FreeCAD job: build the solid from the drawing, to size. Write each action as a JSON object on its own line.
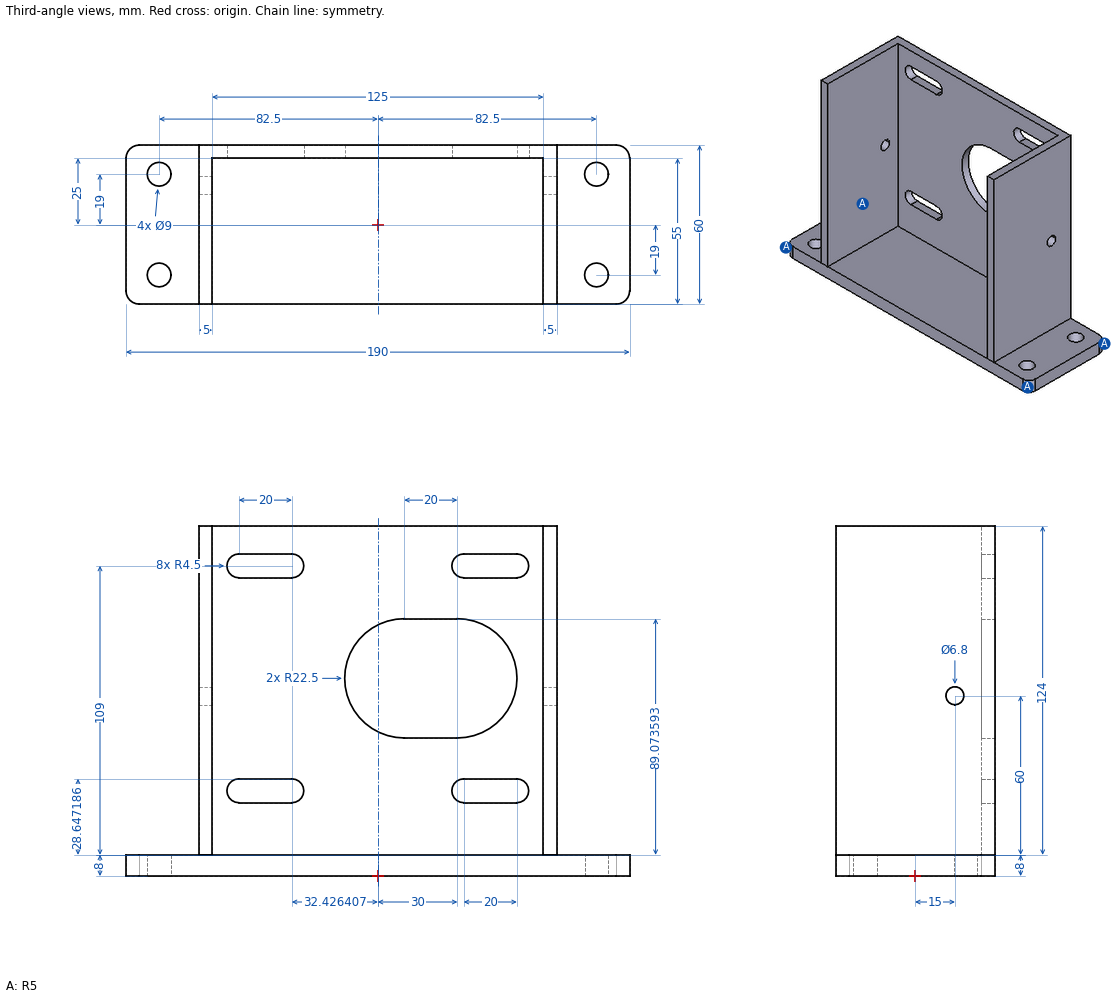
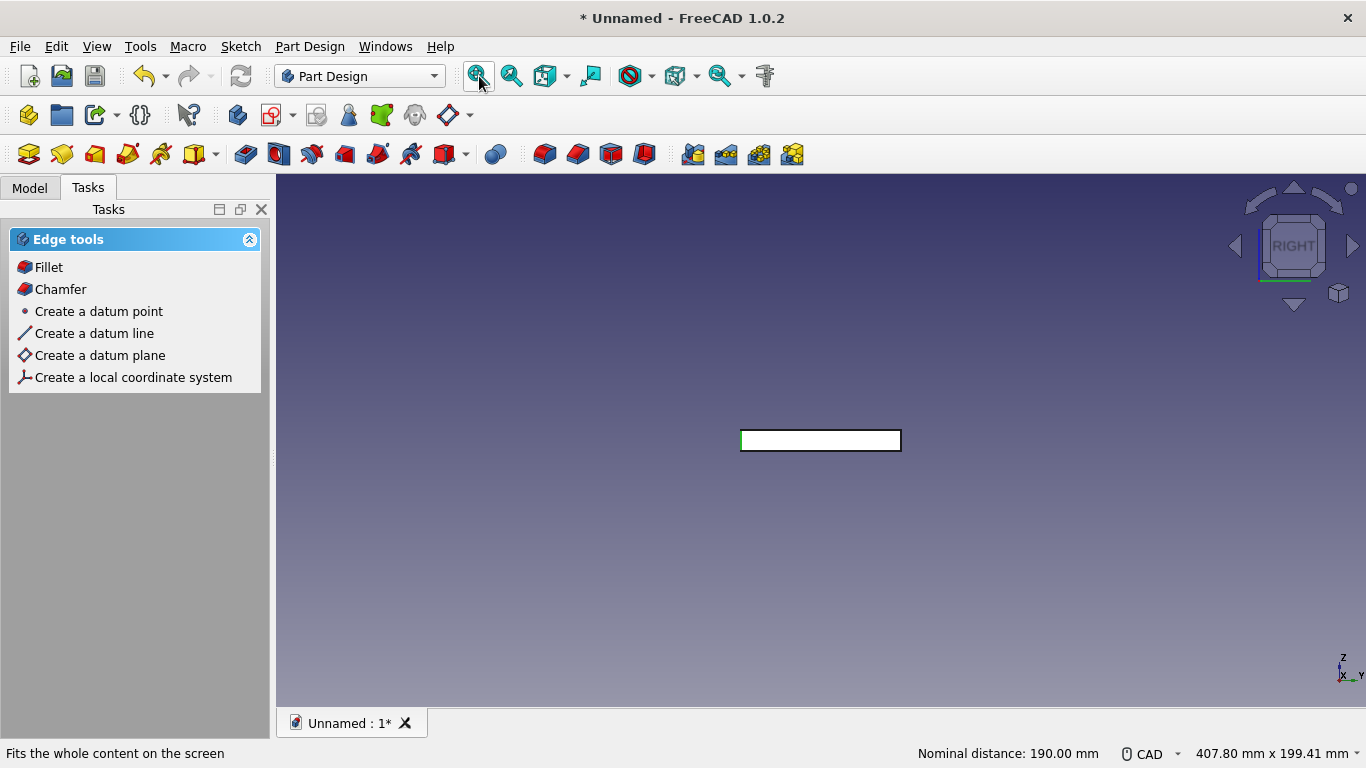
{"action": "left_click", "coordinate": [901, 439], "text": "ctrl"}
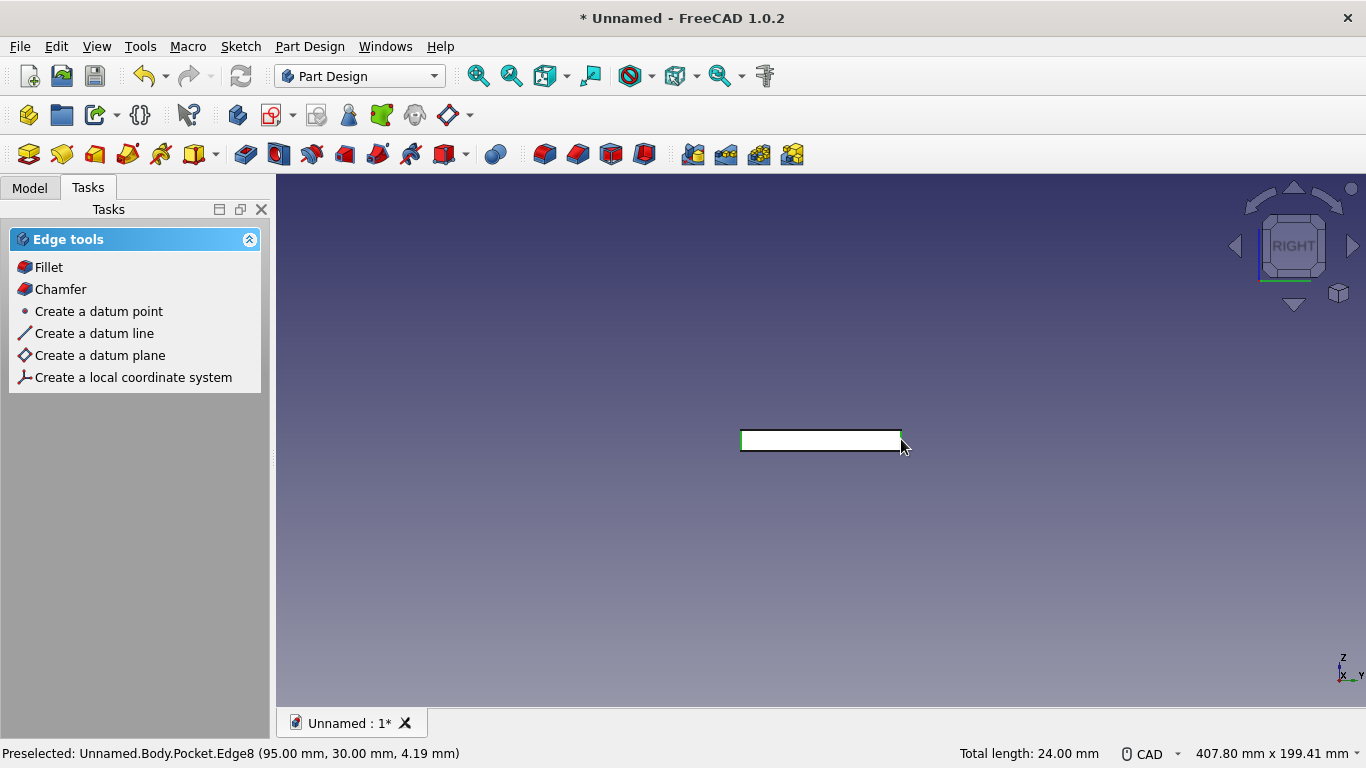
{"action": "scroll", "coordinate": [901, 439], "scroll_direction": "up", "scroll_amount": 4}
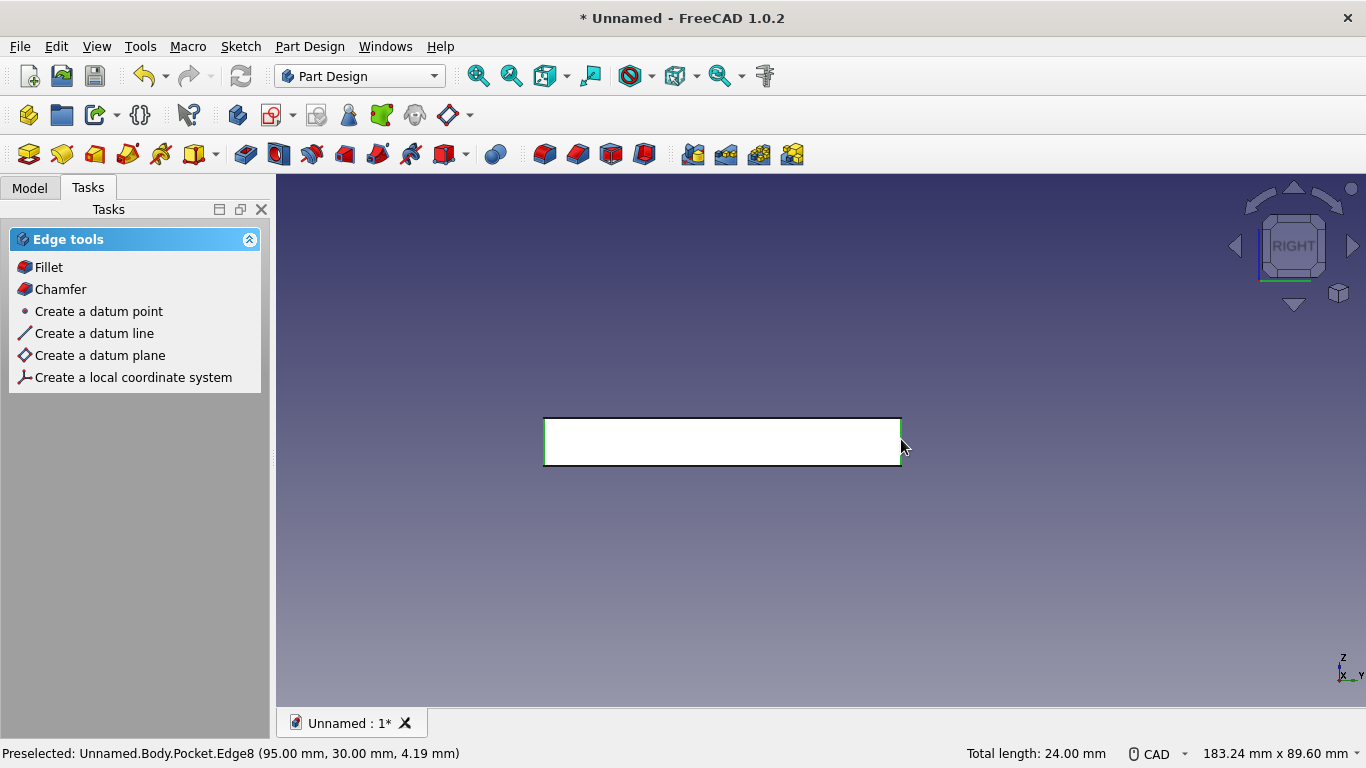
{"action": "left_click", "coordinate": [479, 76]}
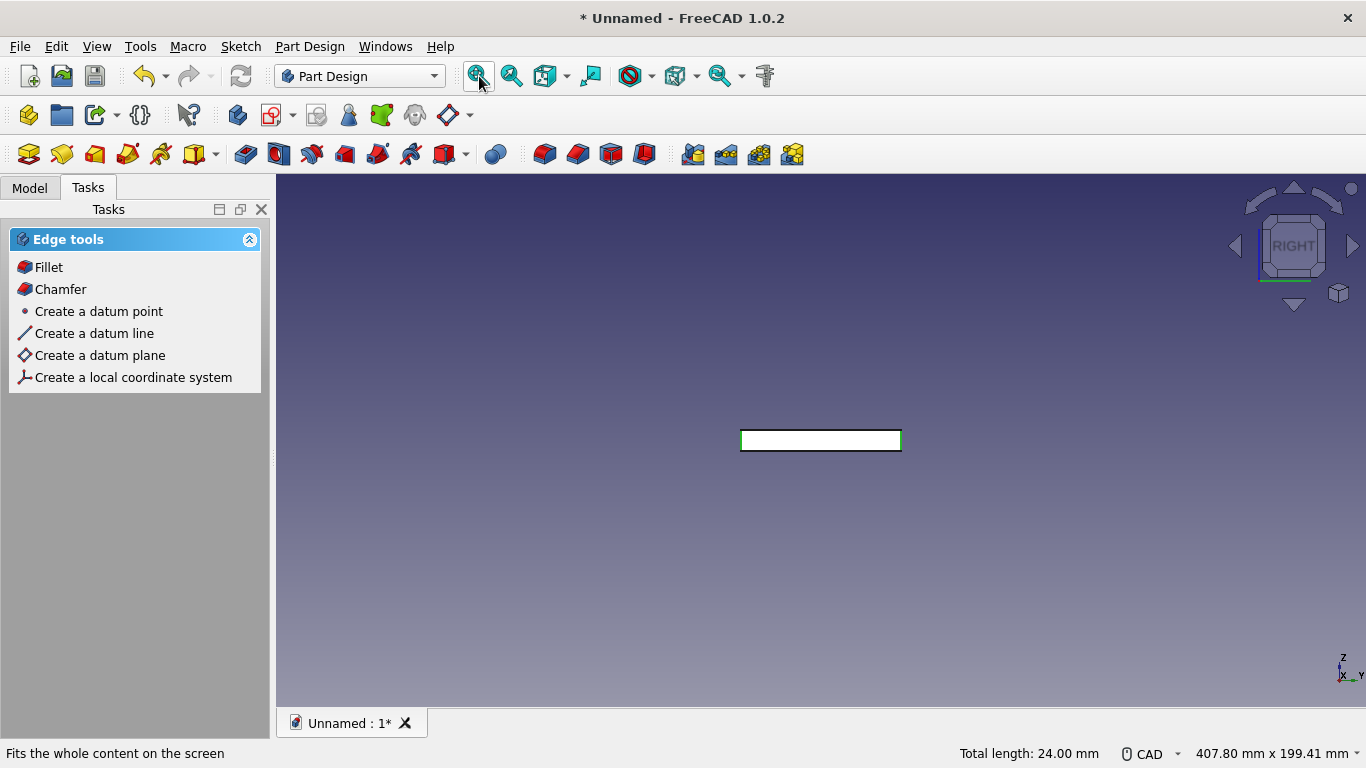
{"action": "key", "text": "5"}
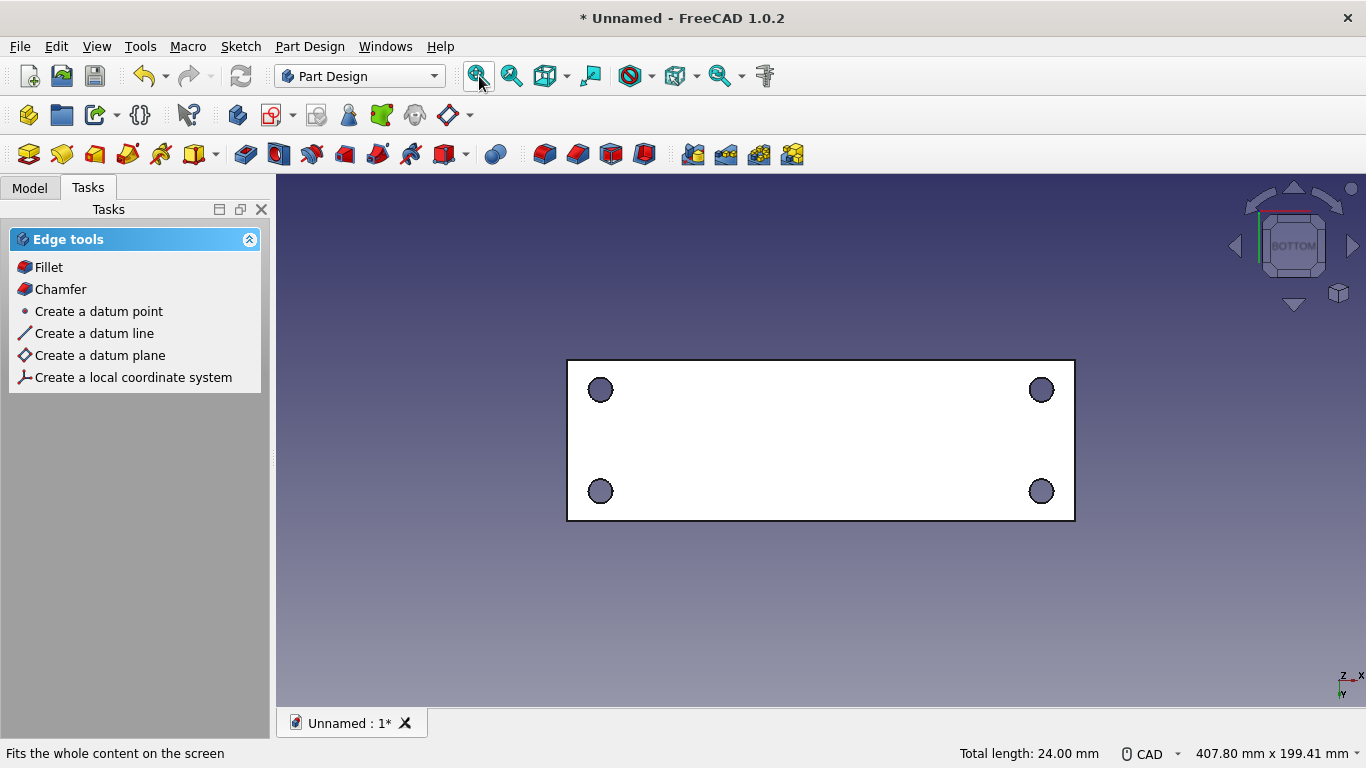
{"action": "scroll", "coordinate": [567, 520], "scroll_direction": "up", "scroll_amount": 4}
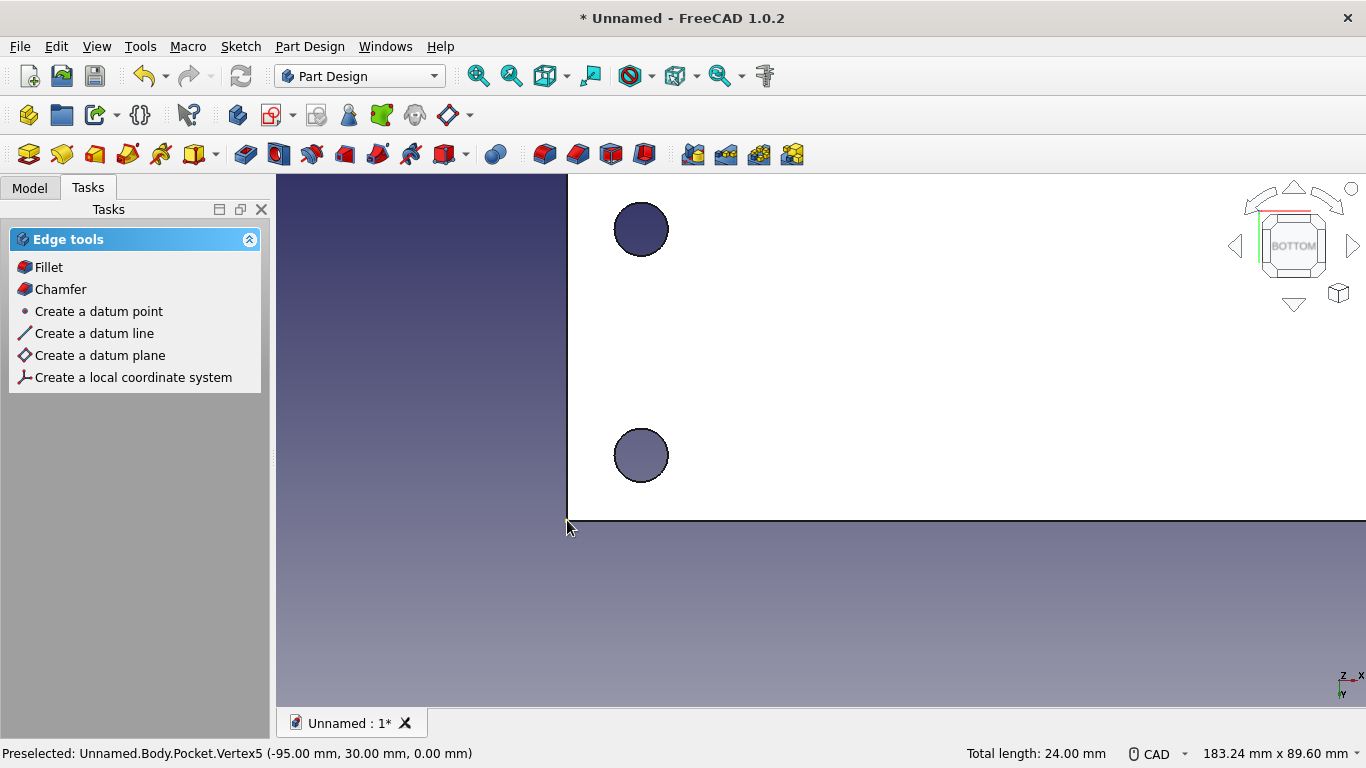
{"action": "left_click", "coordinate": [479, 76]}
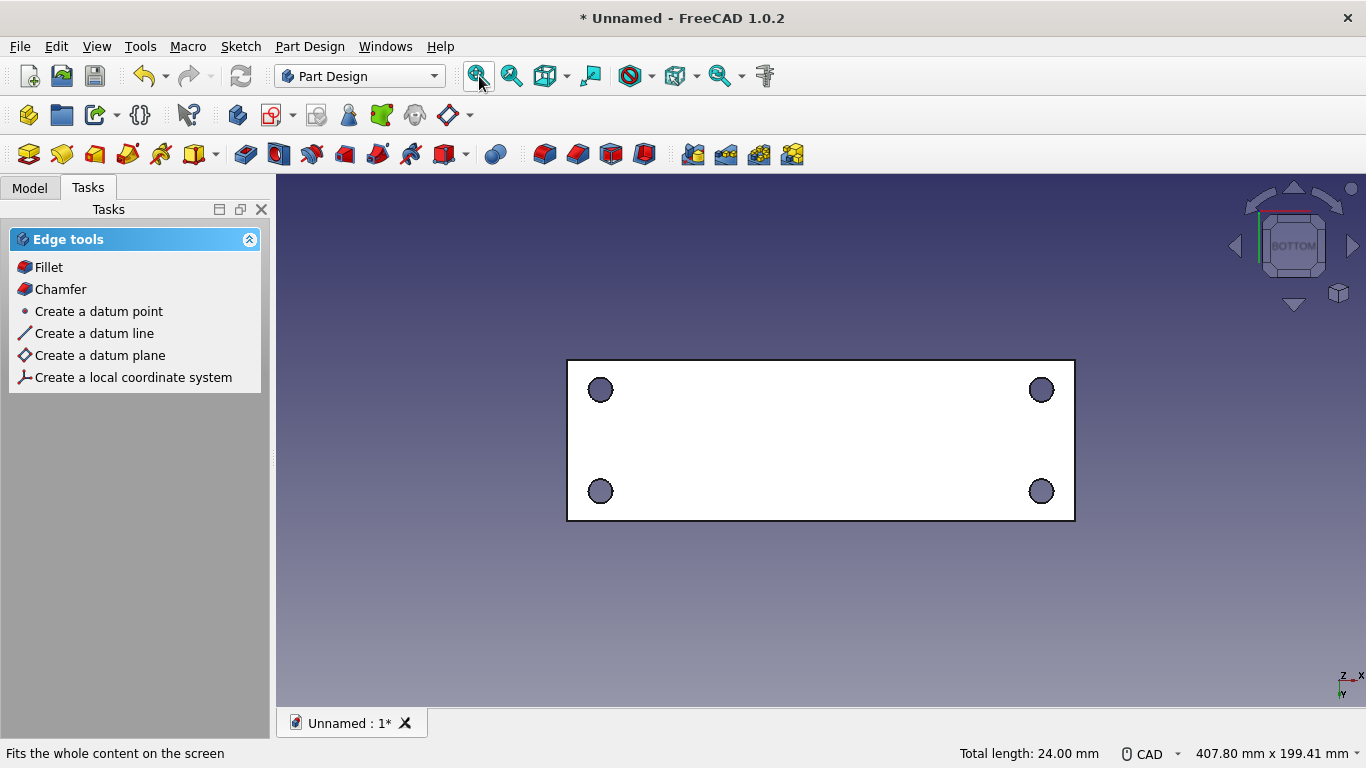
{"action": "key", "text": "4"}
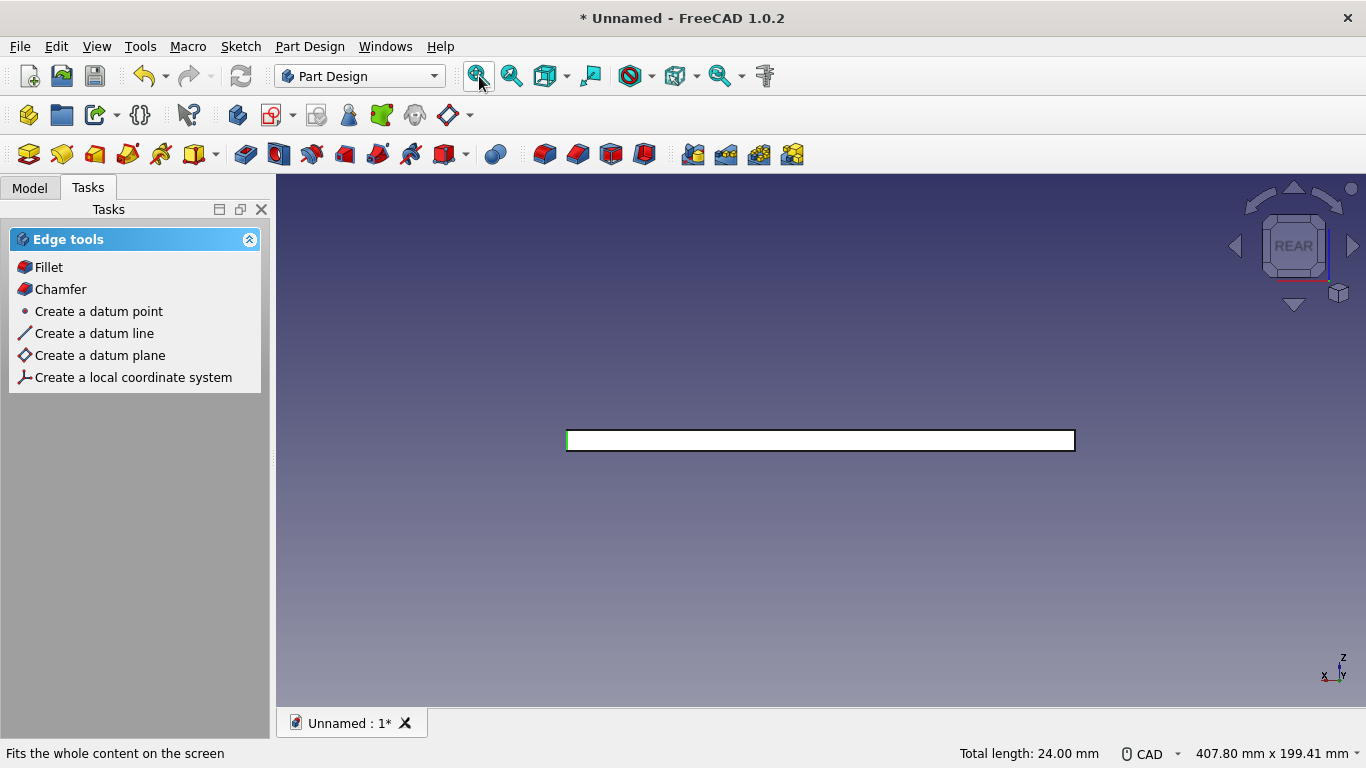
{"action": "left_click", "coordinate": [1075, 439], "text": "ctrl"}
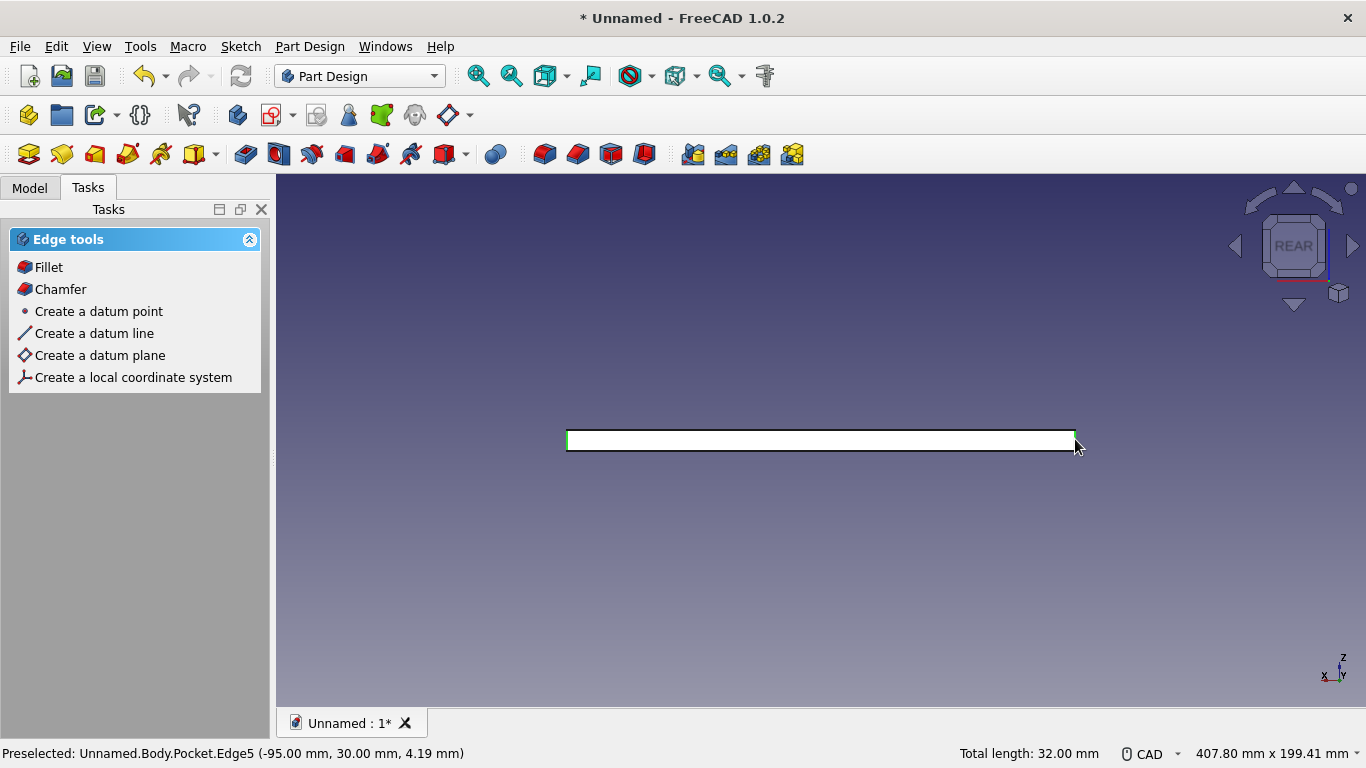
{"action": "left_click", "coordinate": [545, 154]}